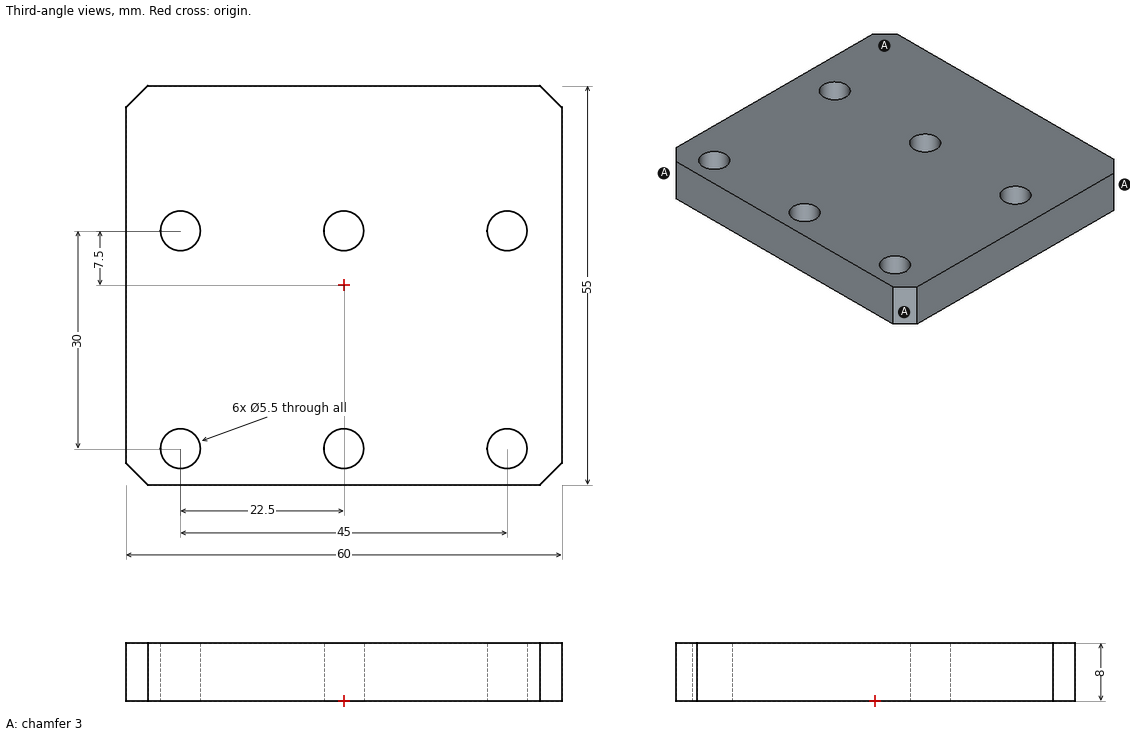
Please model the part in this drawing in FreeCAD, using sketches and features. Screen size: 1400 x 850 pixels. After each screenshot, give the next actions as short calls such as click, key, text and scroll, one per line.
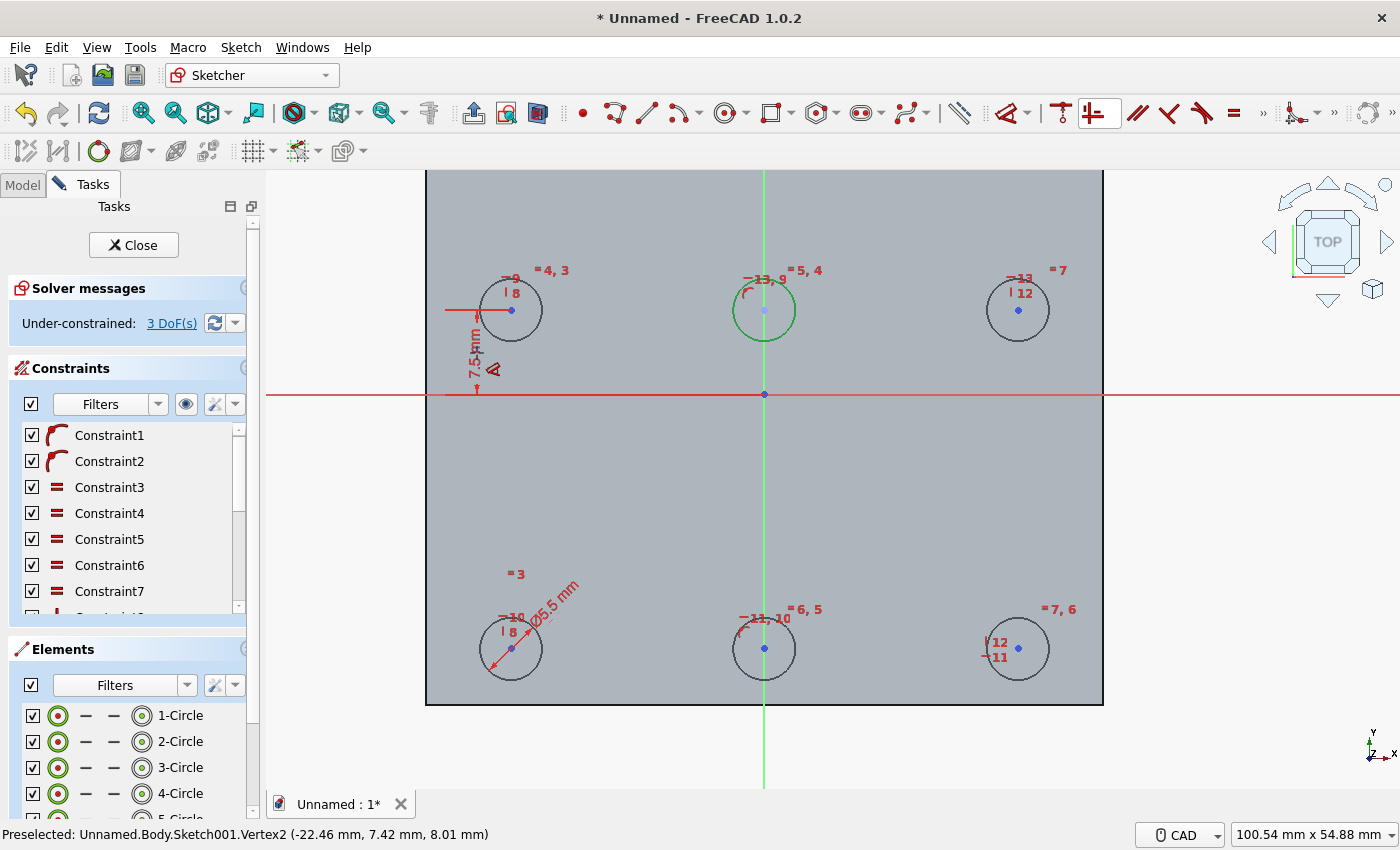
click(511, 649)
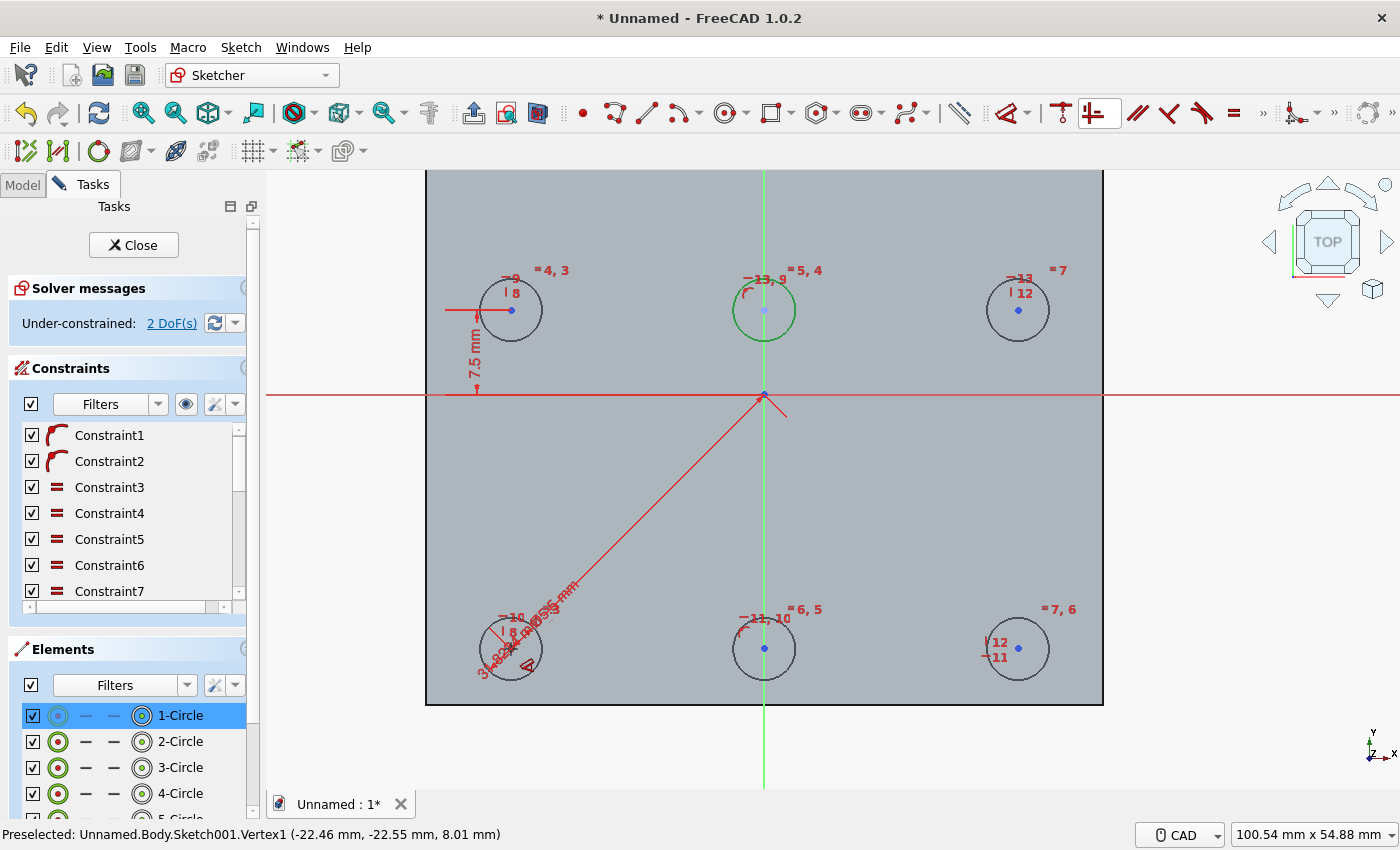
click(511, 310)
click(477, 480)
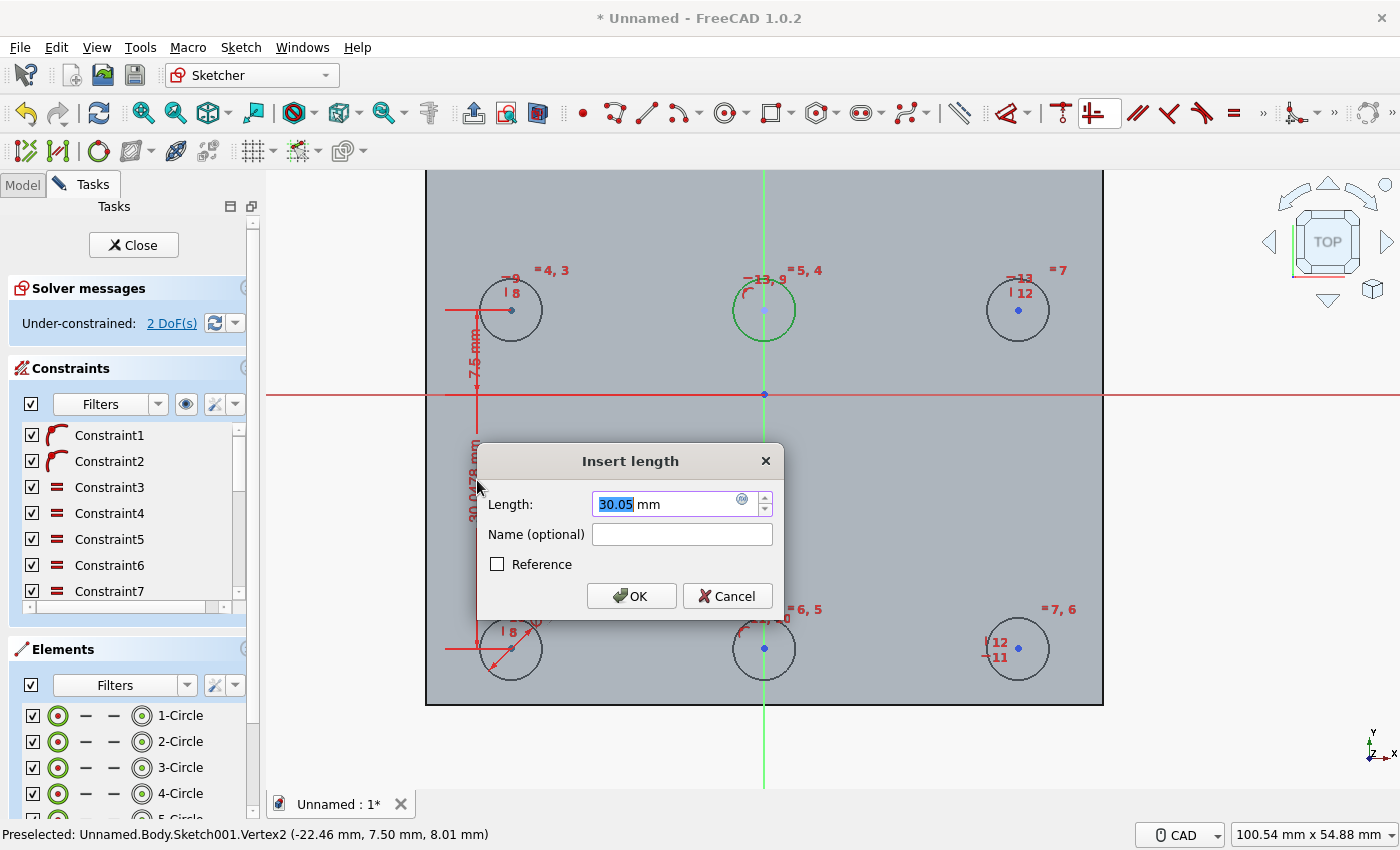
text(30)
key(Return)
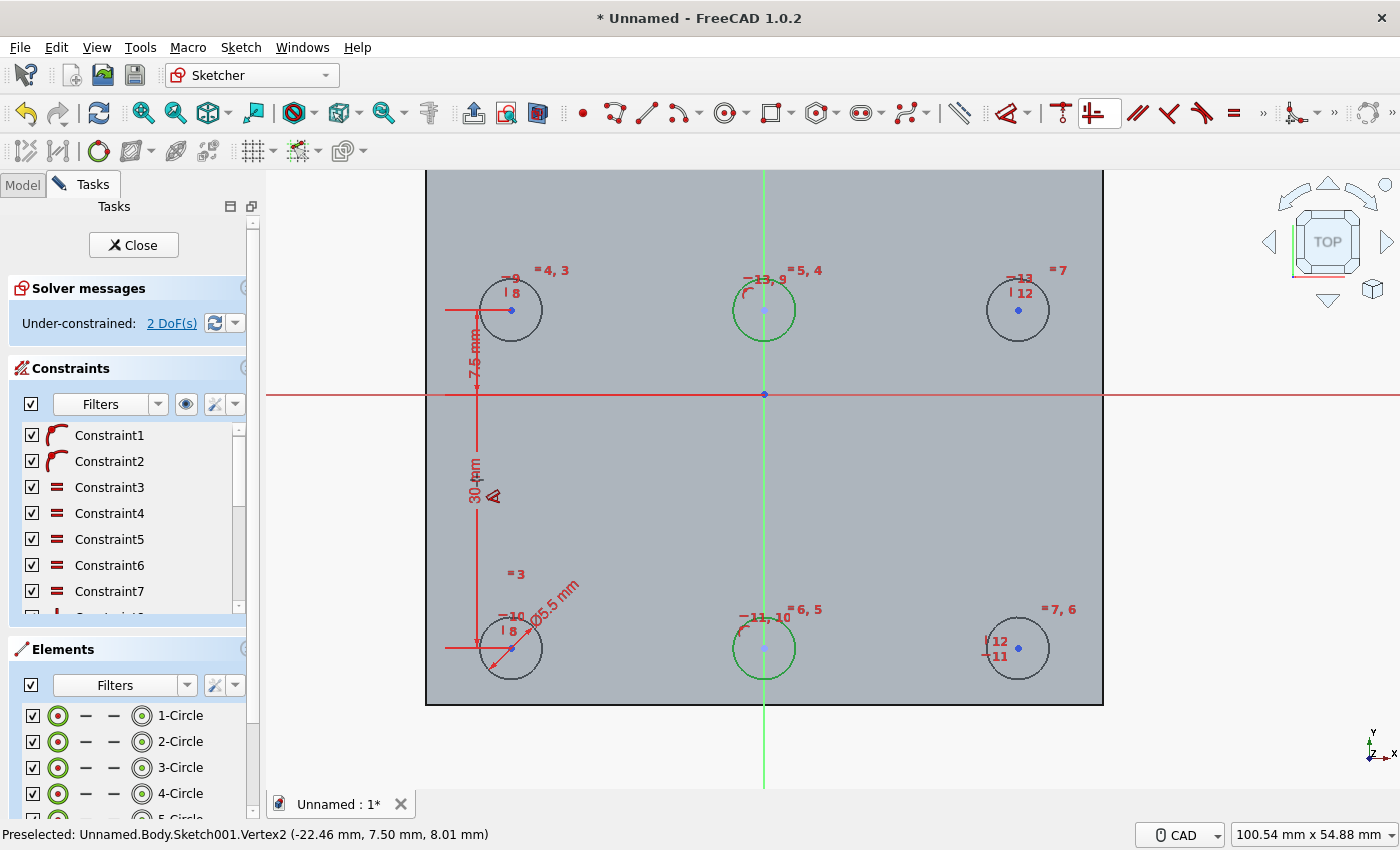
click(511, 648)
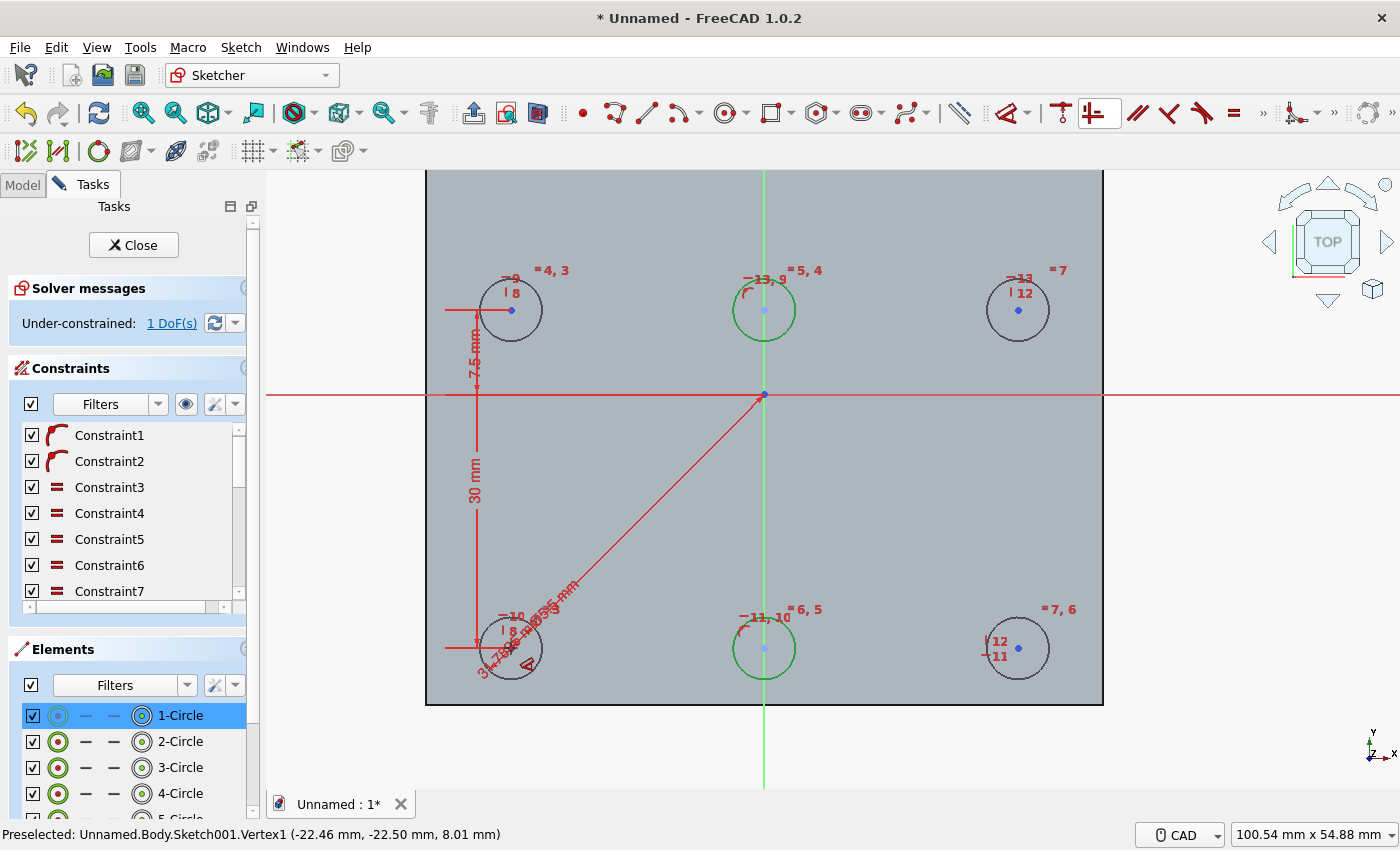
click(1018, 648)
click(648, 682)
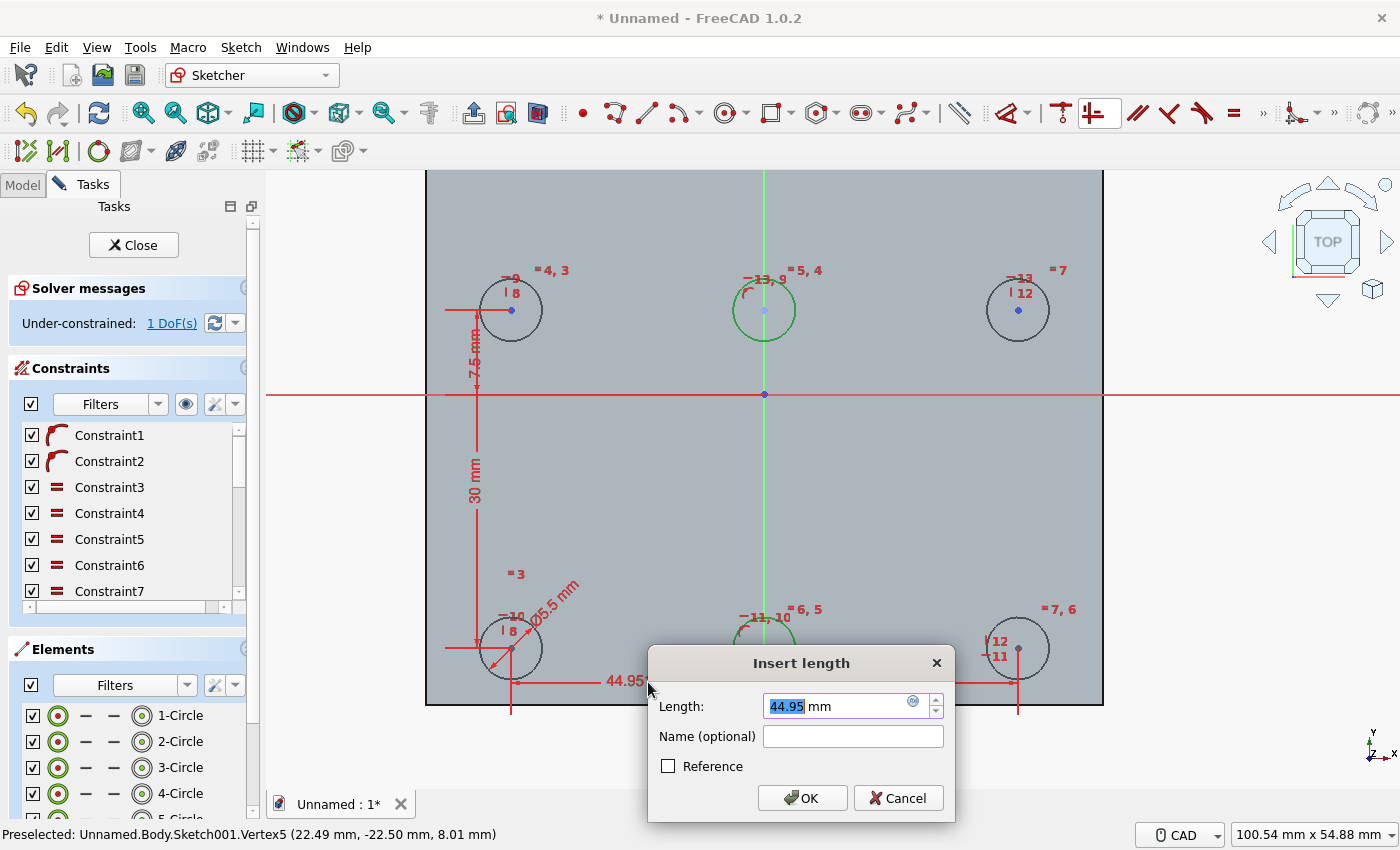
text(45)
key(Return)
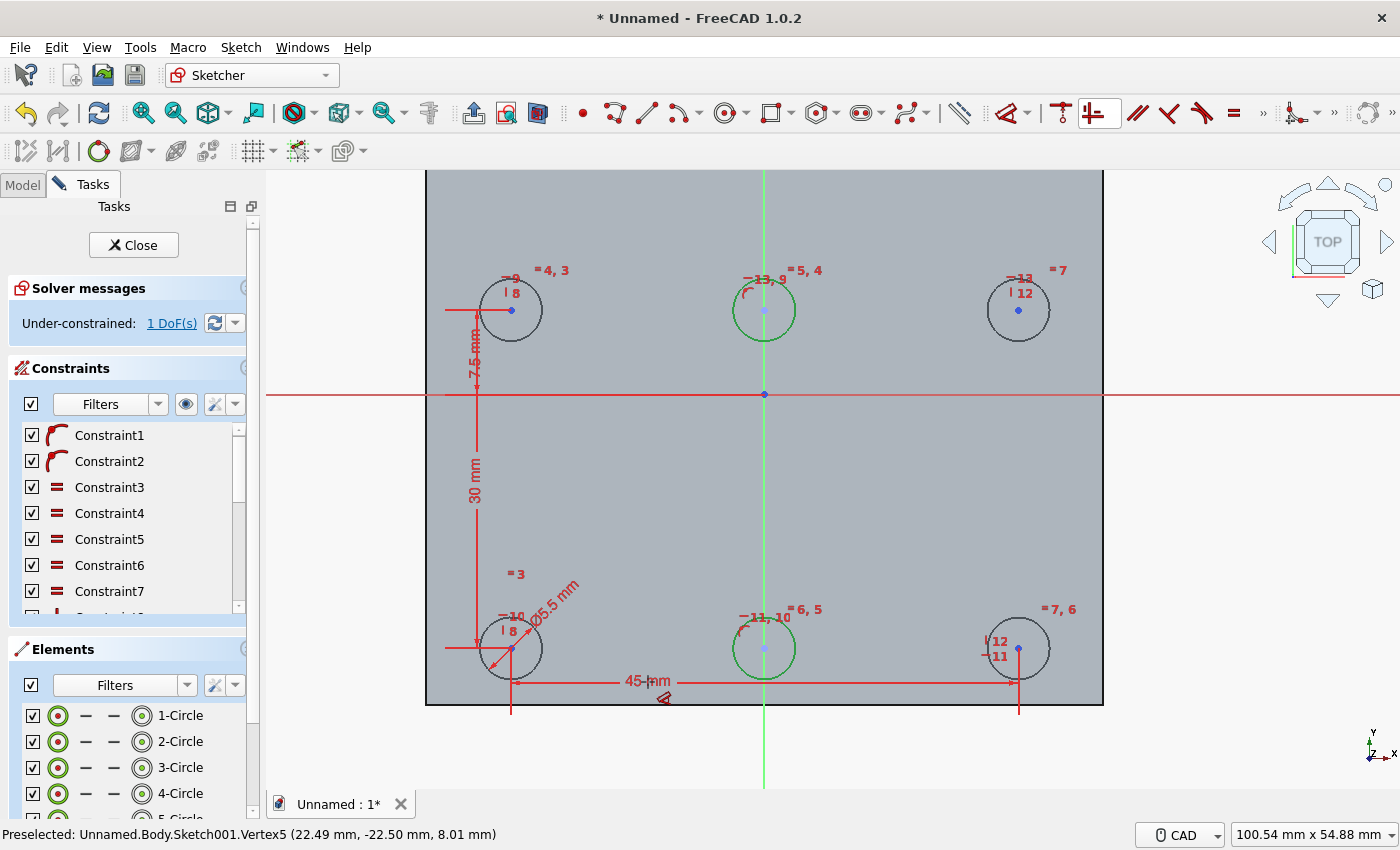
click(511, 648)
click(549, 682)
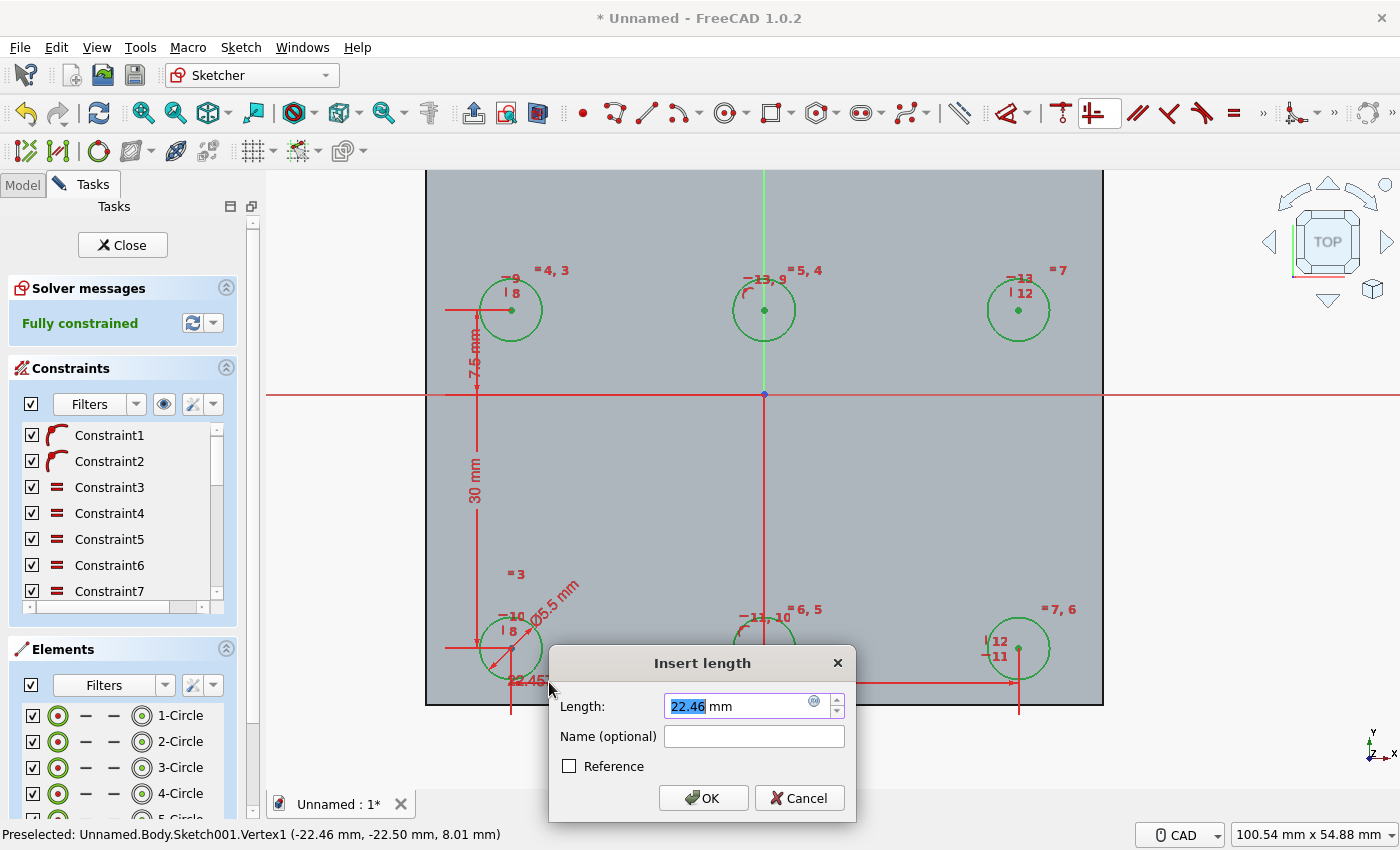
text(22.5)
key(Return)
key(Escape)